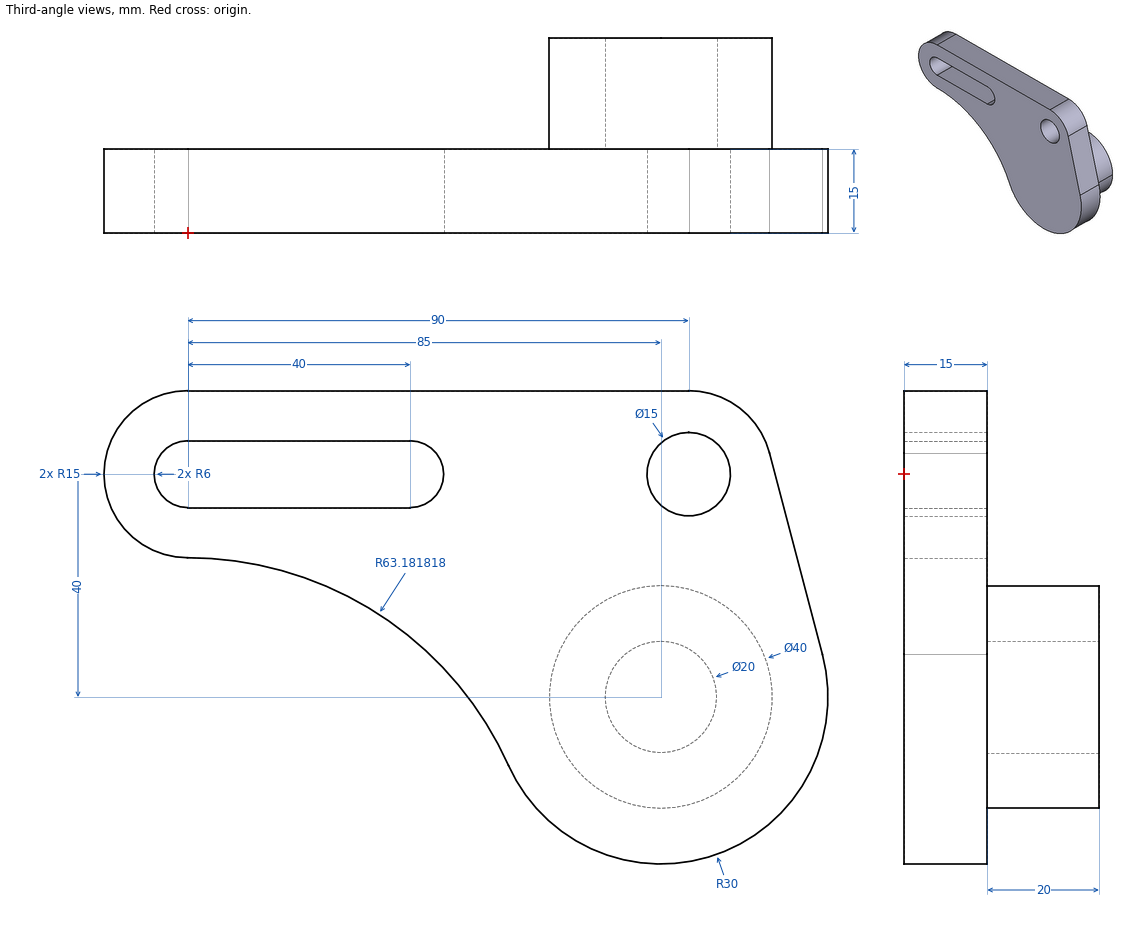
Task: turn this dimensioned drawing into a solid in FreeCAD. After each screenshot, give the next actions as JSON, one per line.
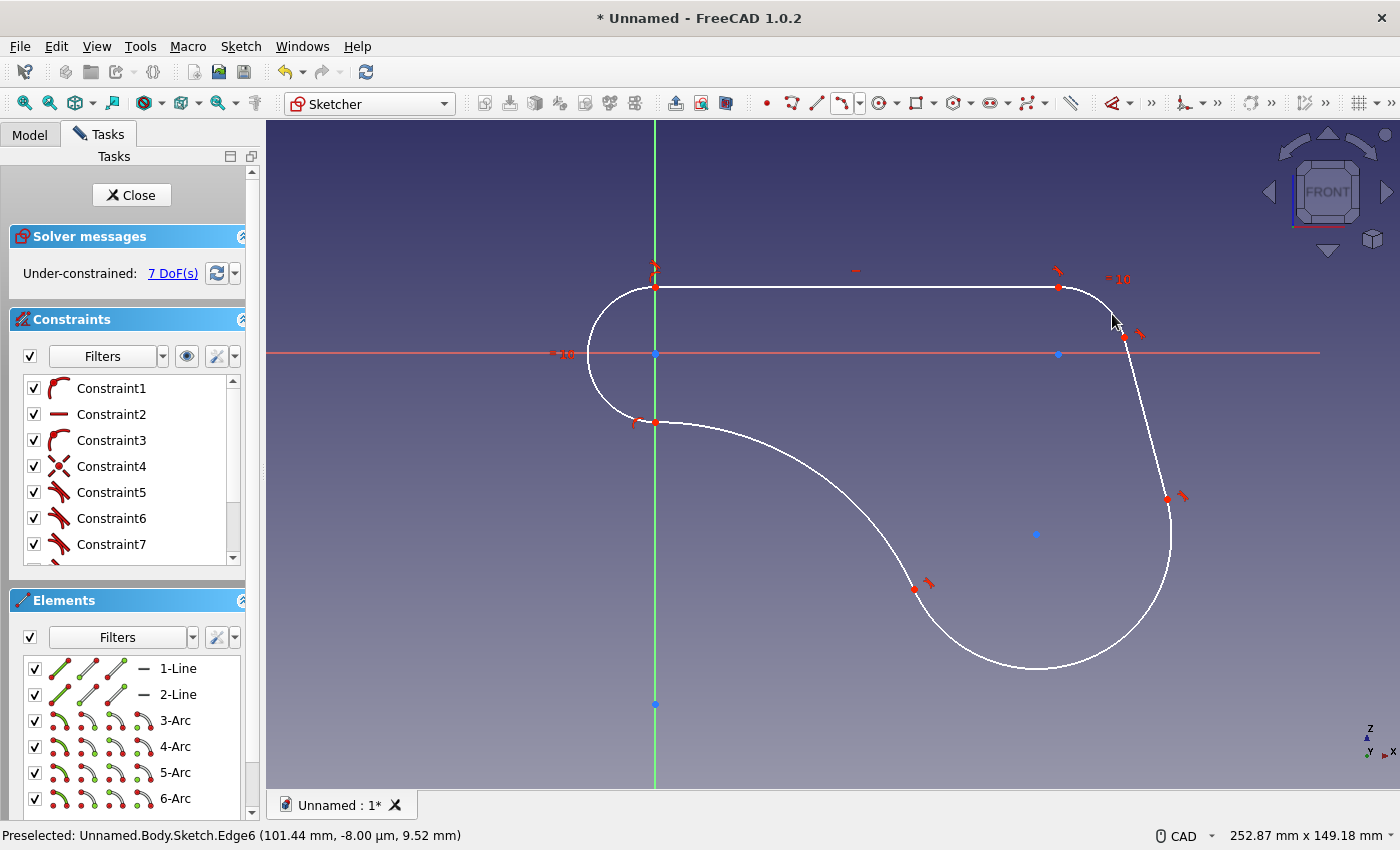
{"action": "left_click", "coordinate": [656, 705]}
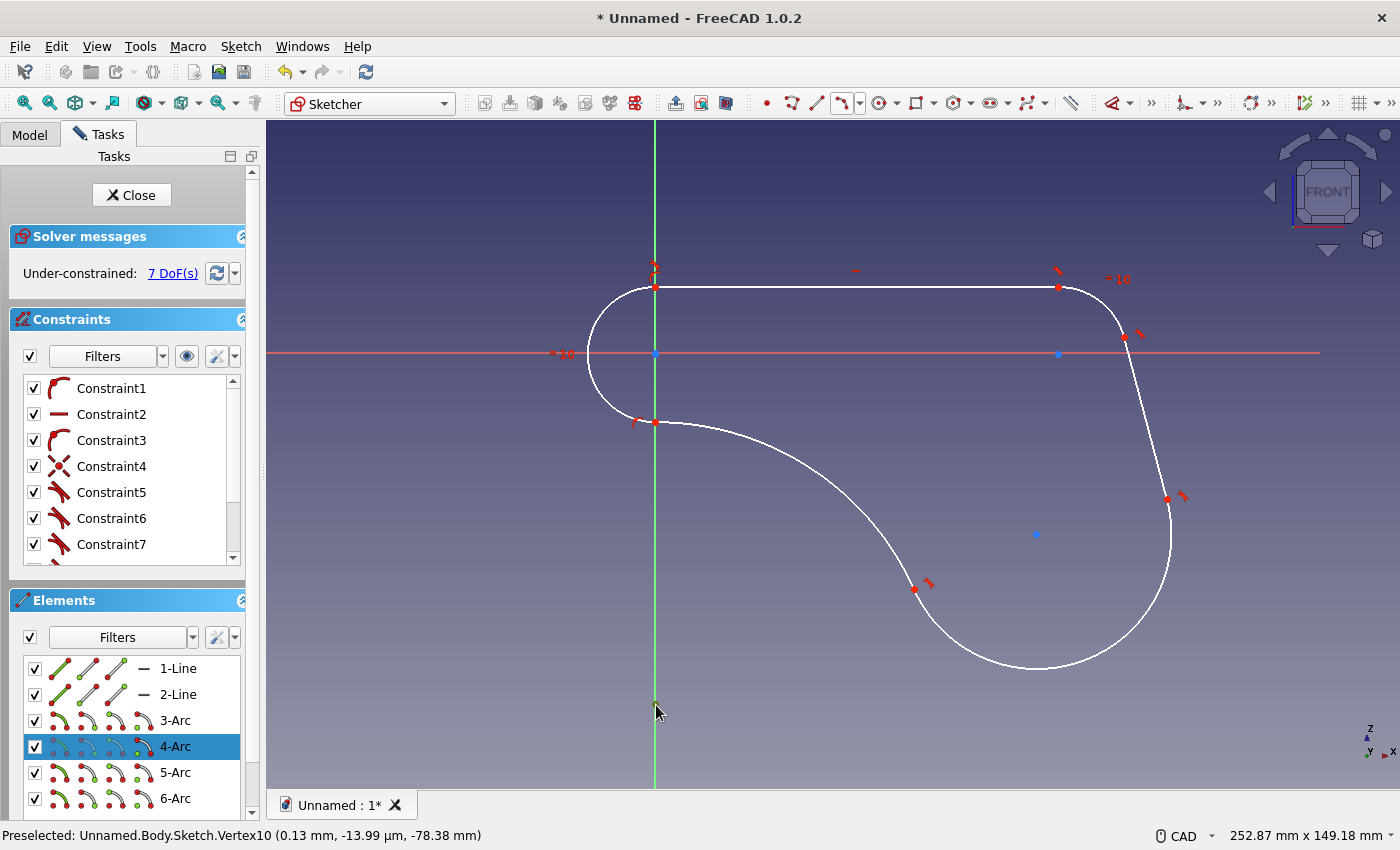
{"action": "left_click", "coordinate": [655, 717]}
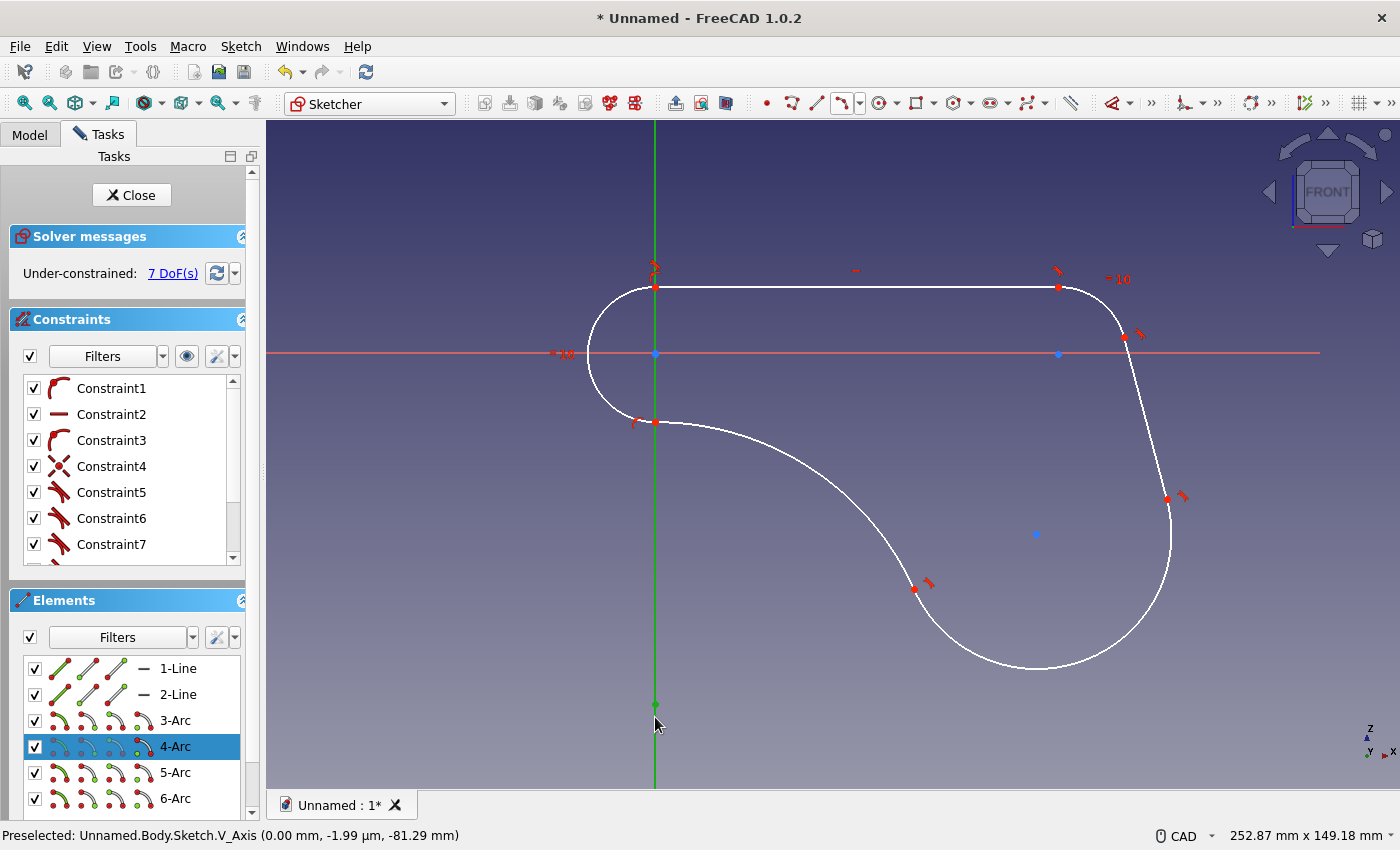
{"action": "key", "text": "c"}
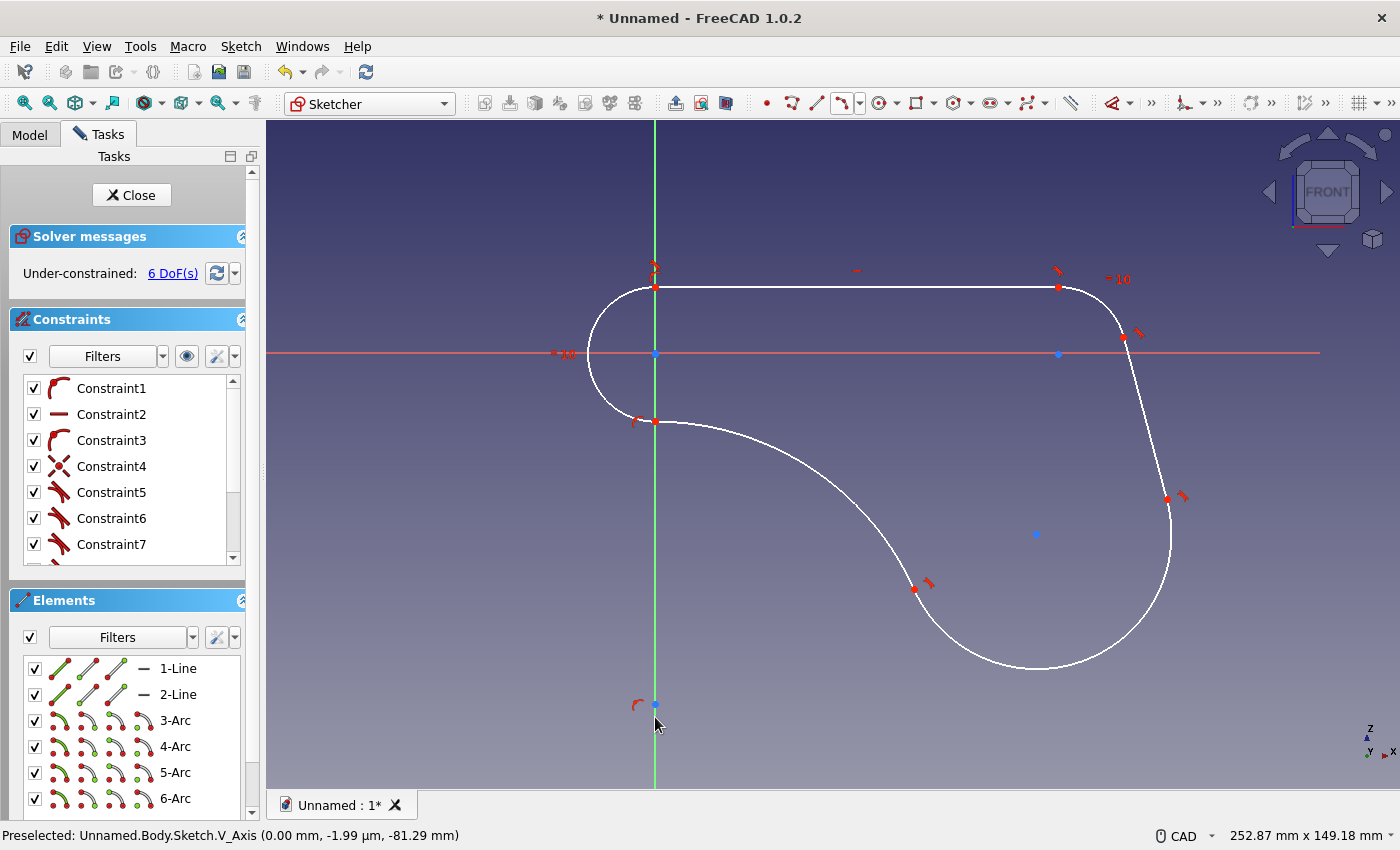
{"action": "left_click", "coordinate": [655, 354]}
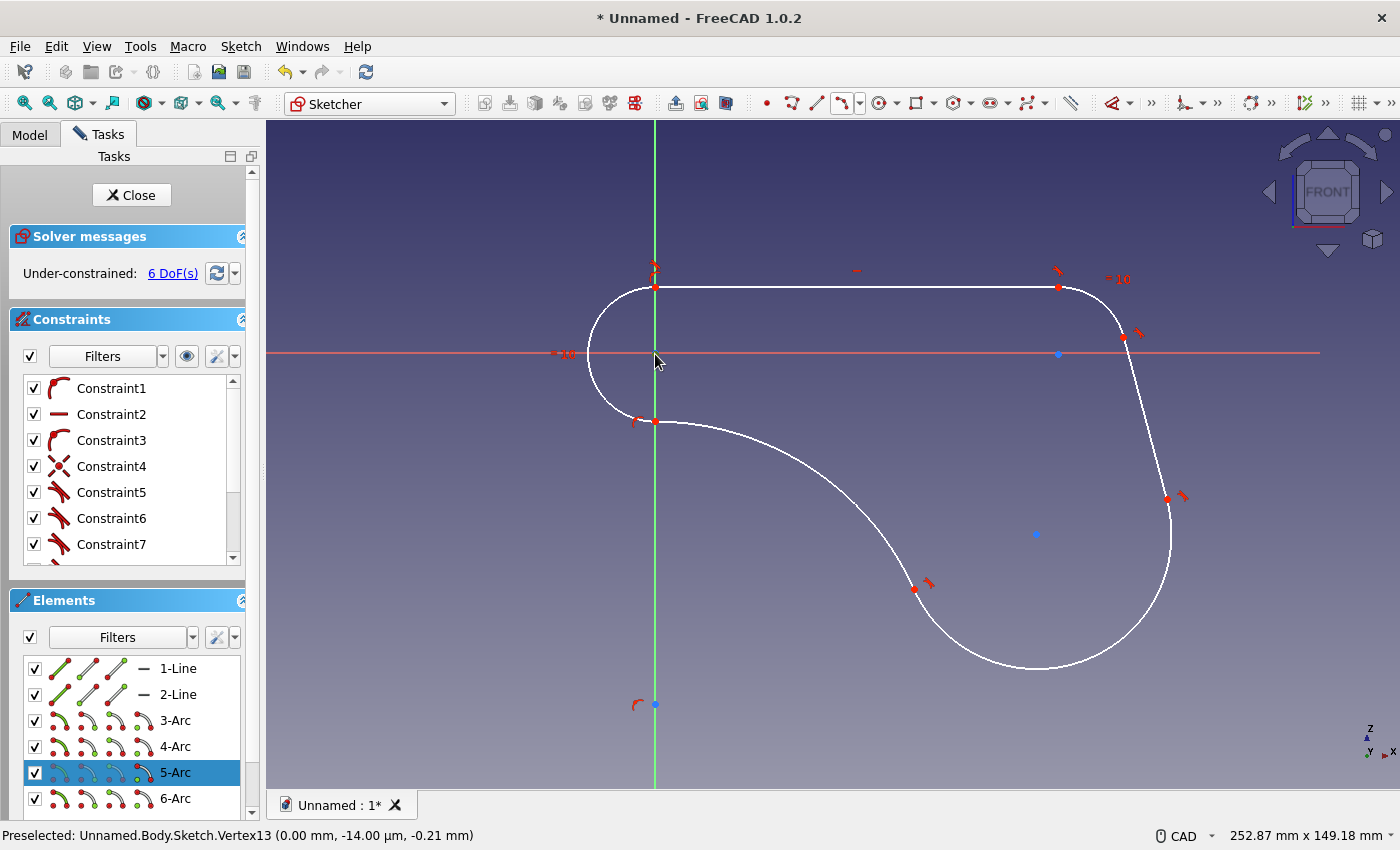
{"action": "left_click", "coordinate": [361, 353]}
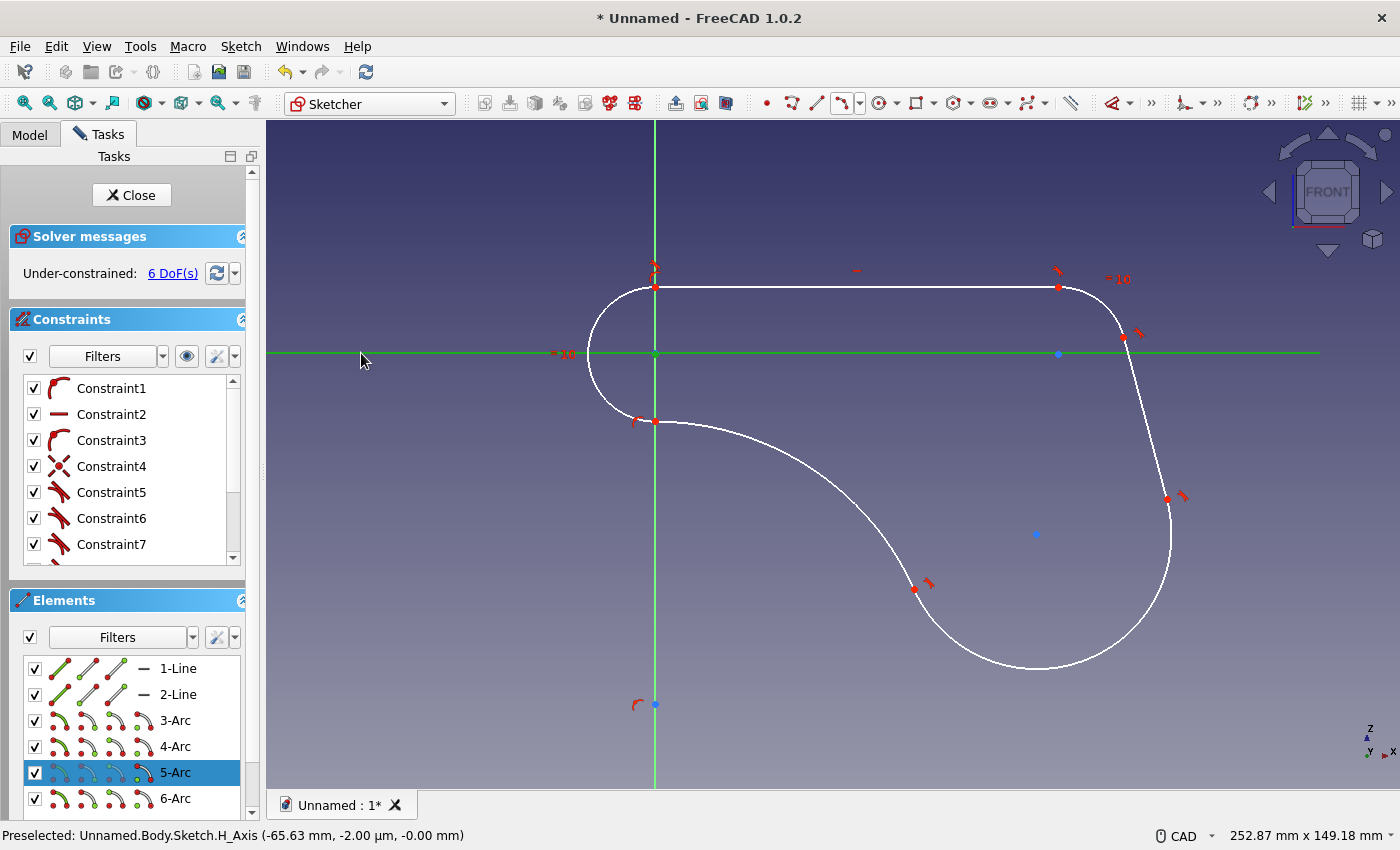
{"action": "key", "text": "c"}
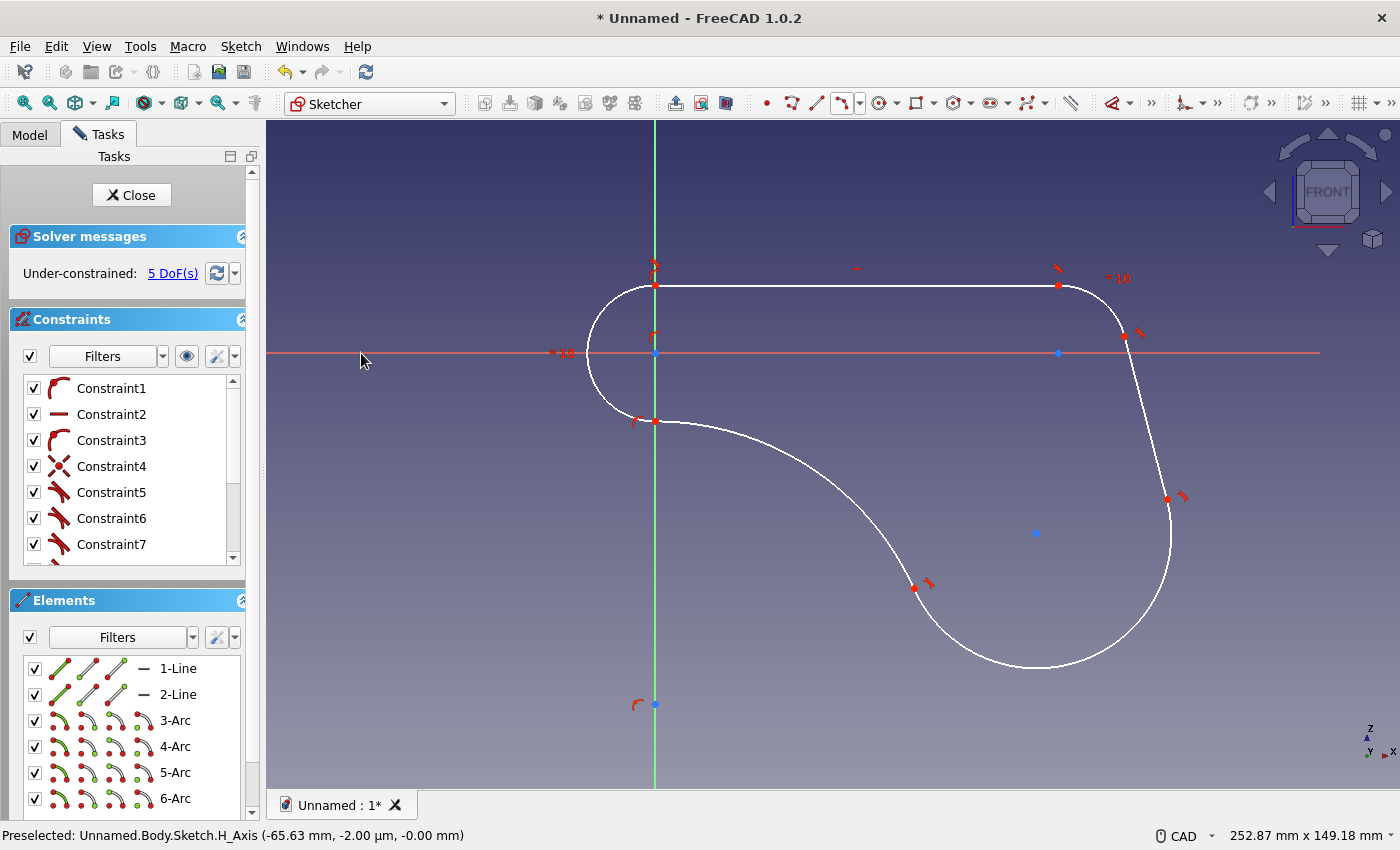
{"action": "left_click", "coordinate": [1003, 664]}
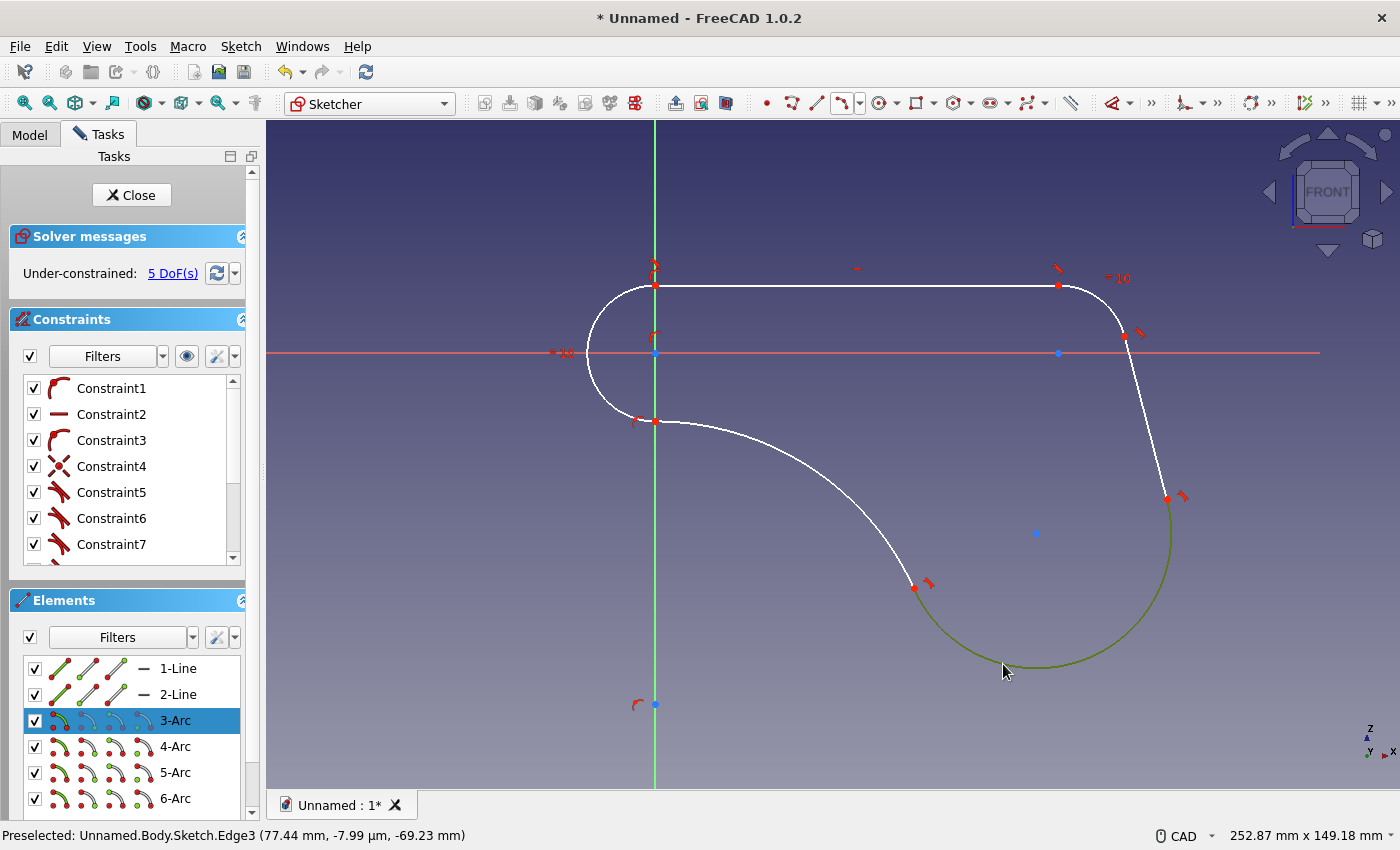
{"action": "key", "text": "k r"}